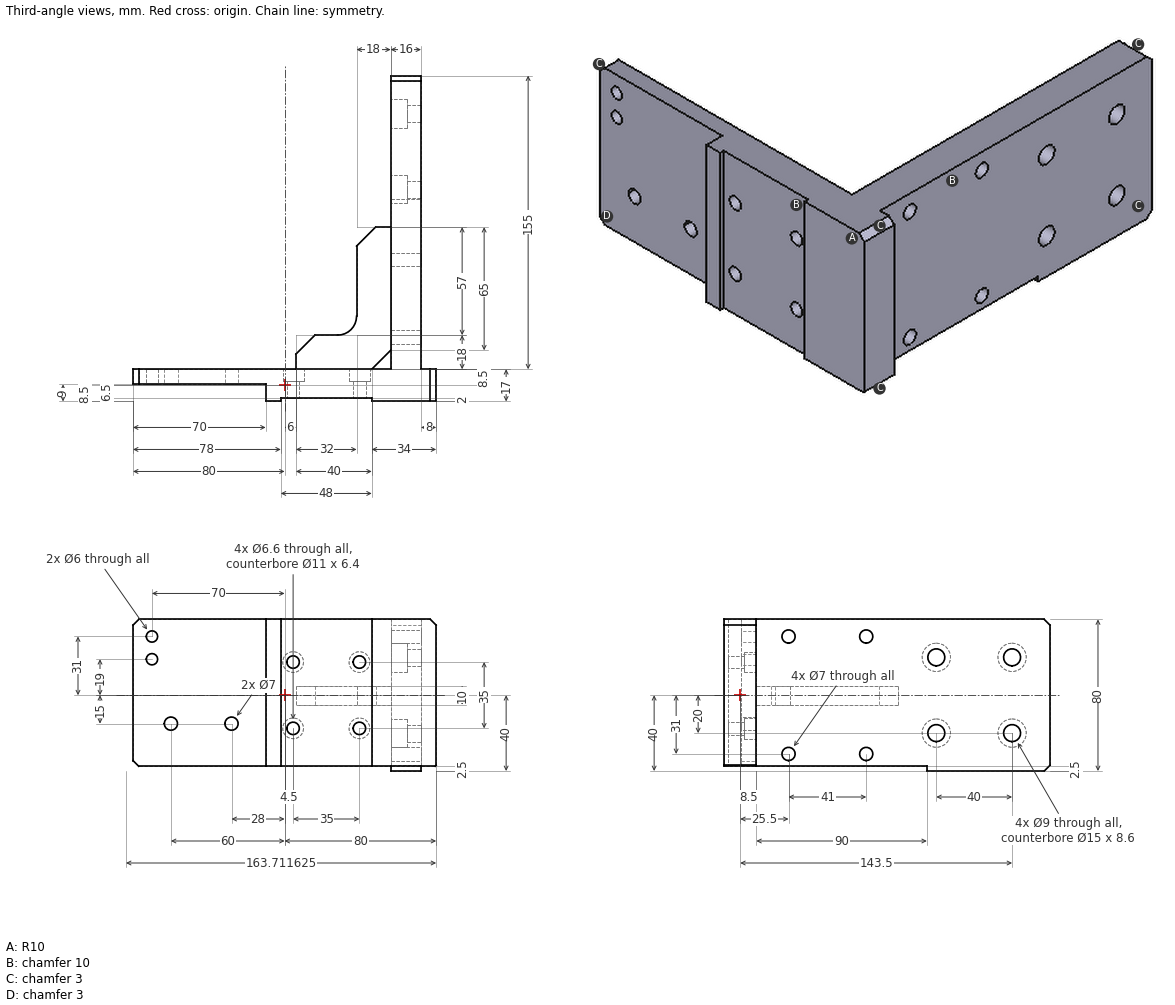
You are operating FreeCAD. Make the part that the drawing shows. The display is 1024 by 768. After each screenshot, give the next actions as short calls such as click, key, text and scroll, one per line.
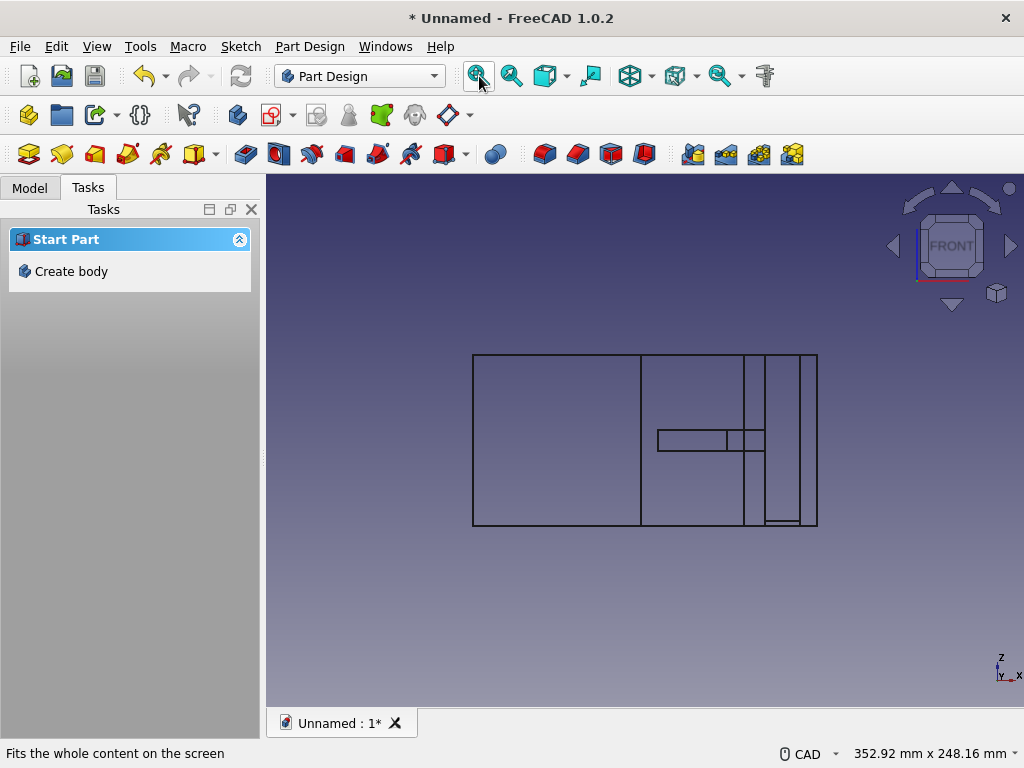
click(727, 440)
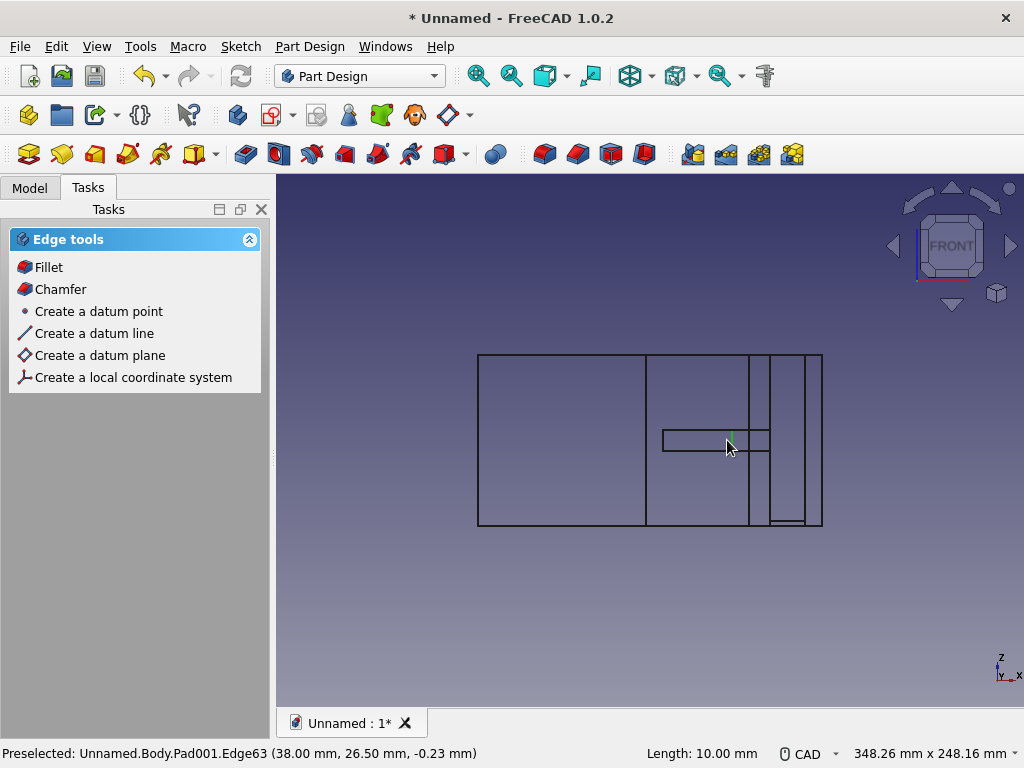
key(v)
key(1)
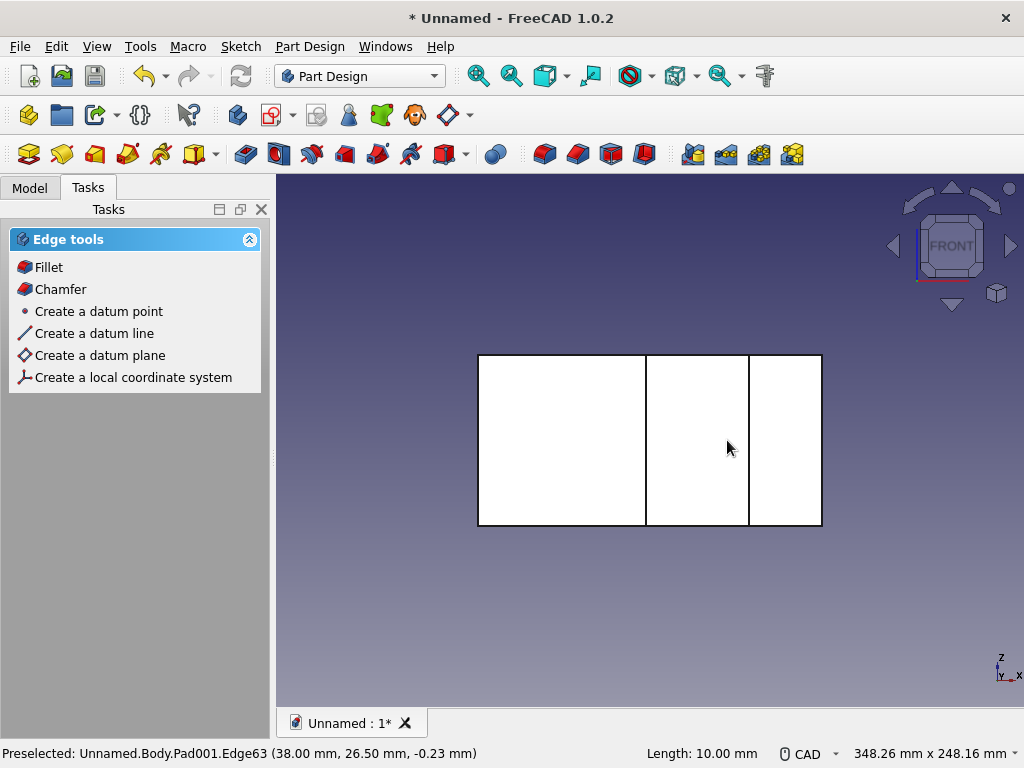
click(545, 154)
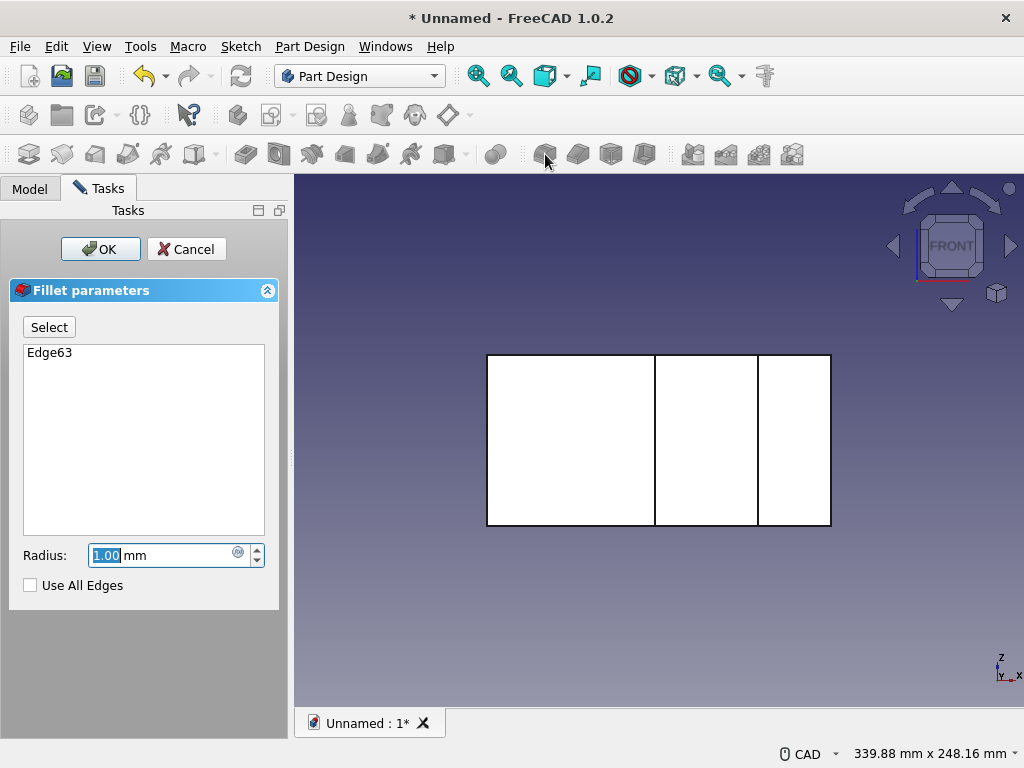
text(10)
key(Tab)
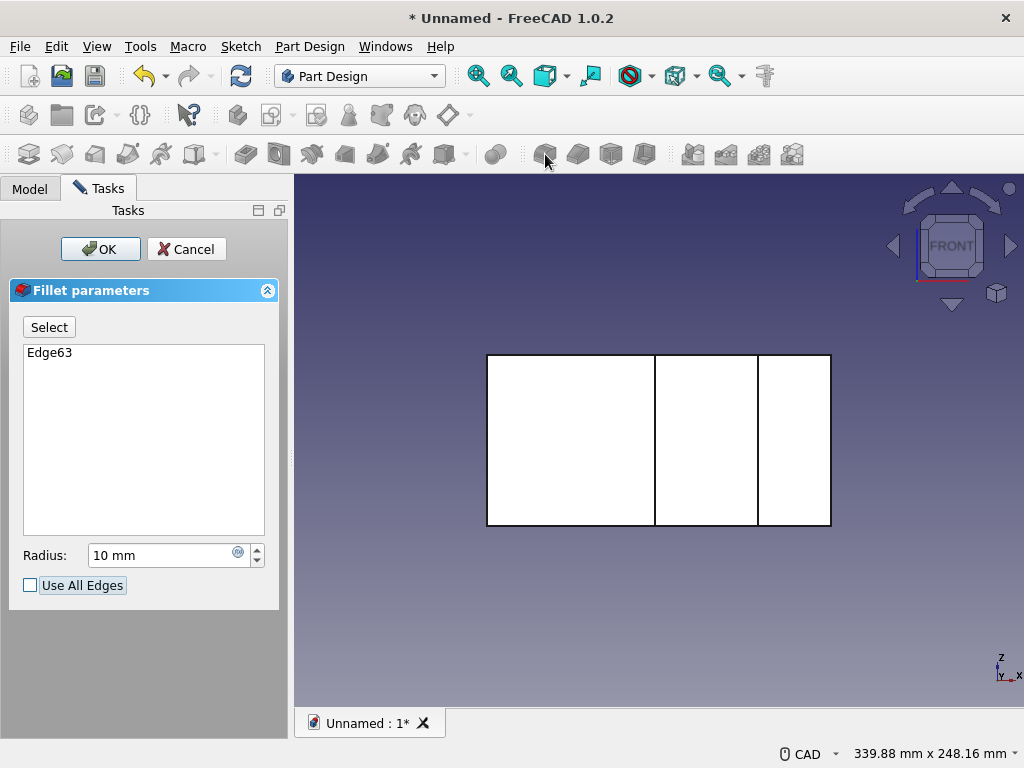
click(101, 249)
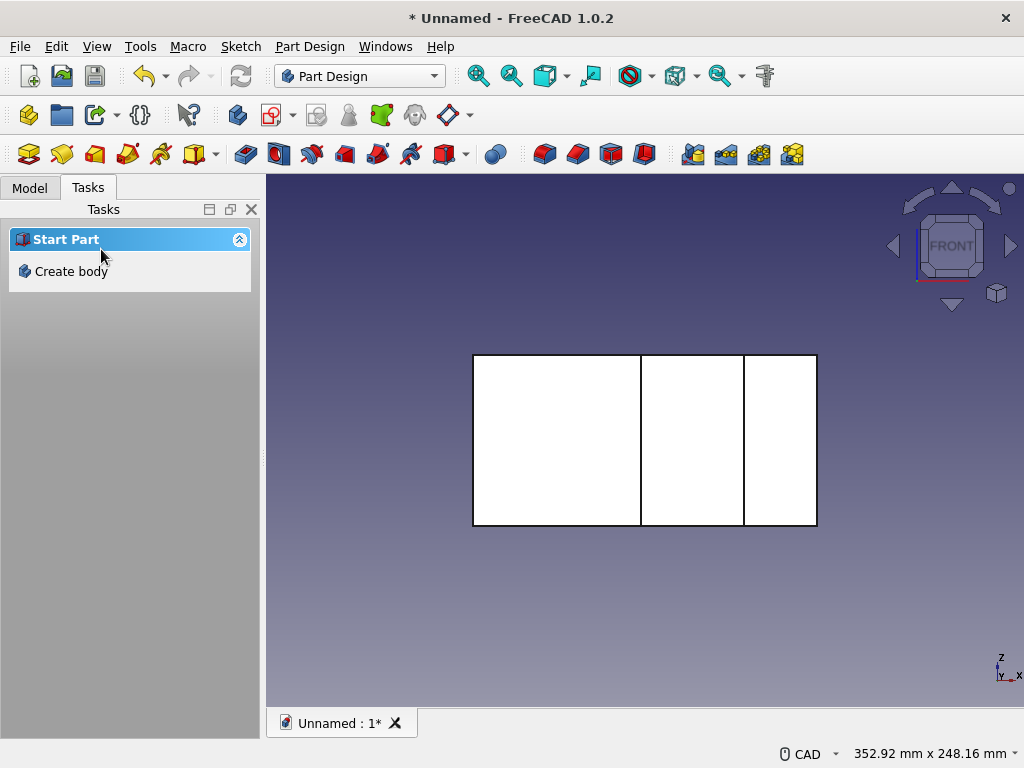
scroll(658, 440, up, 4)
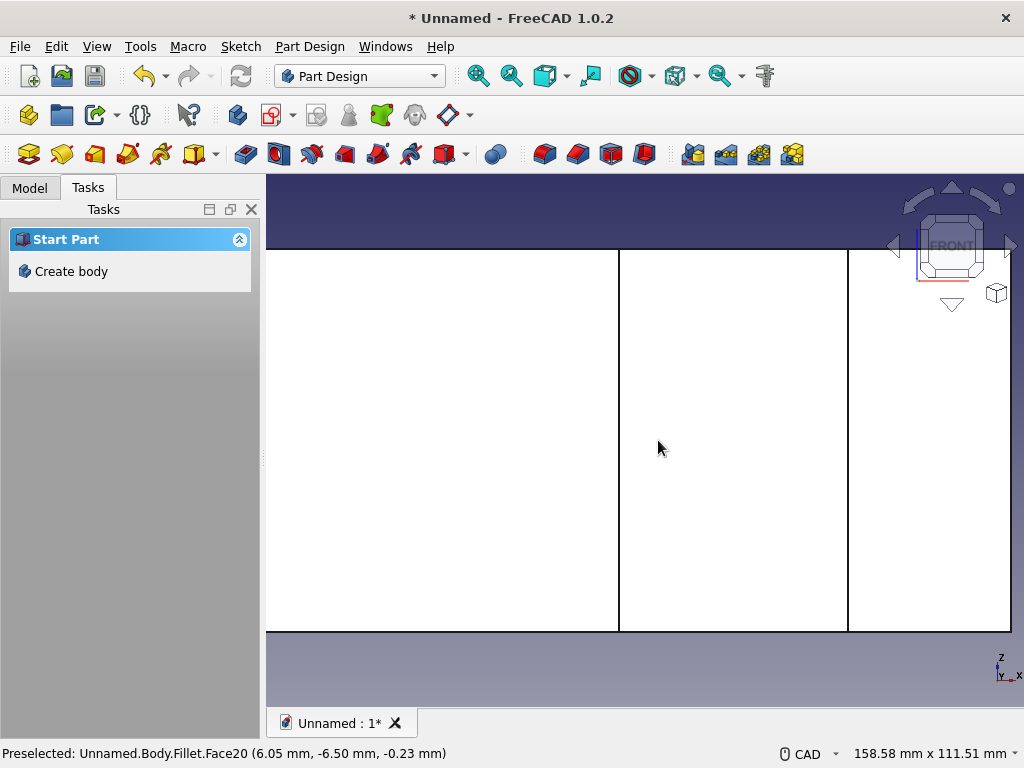
click(479, 76)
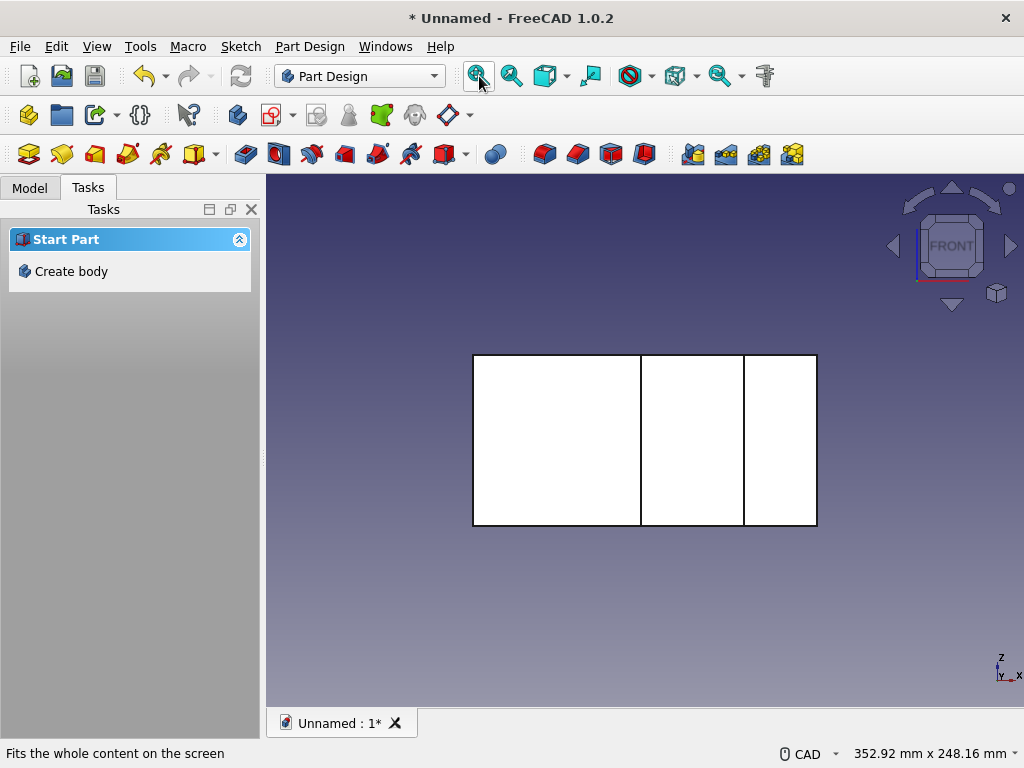
key(0)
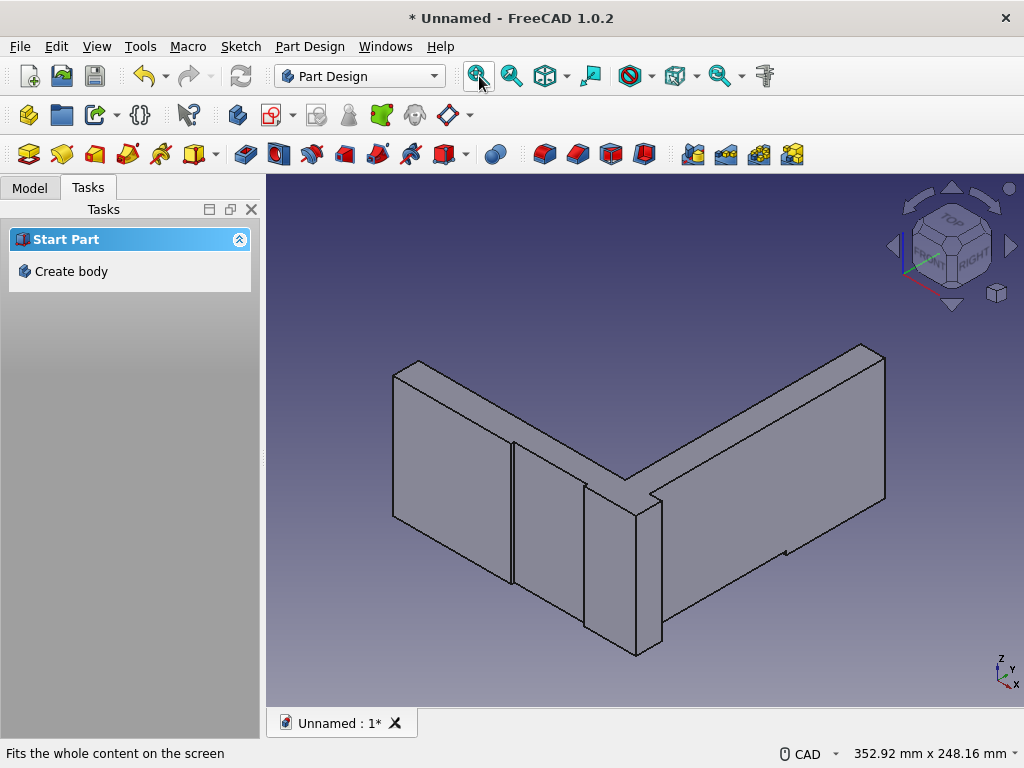
scroll(577, 489, up, 4)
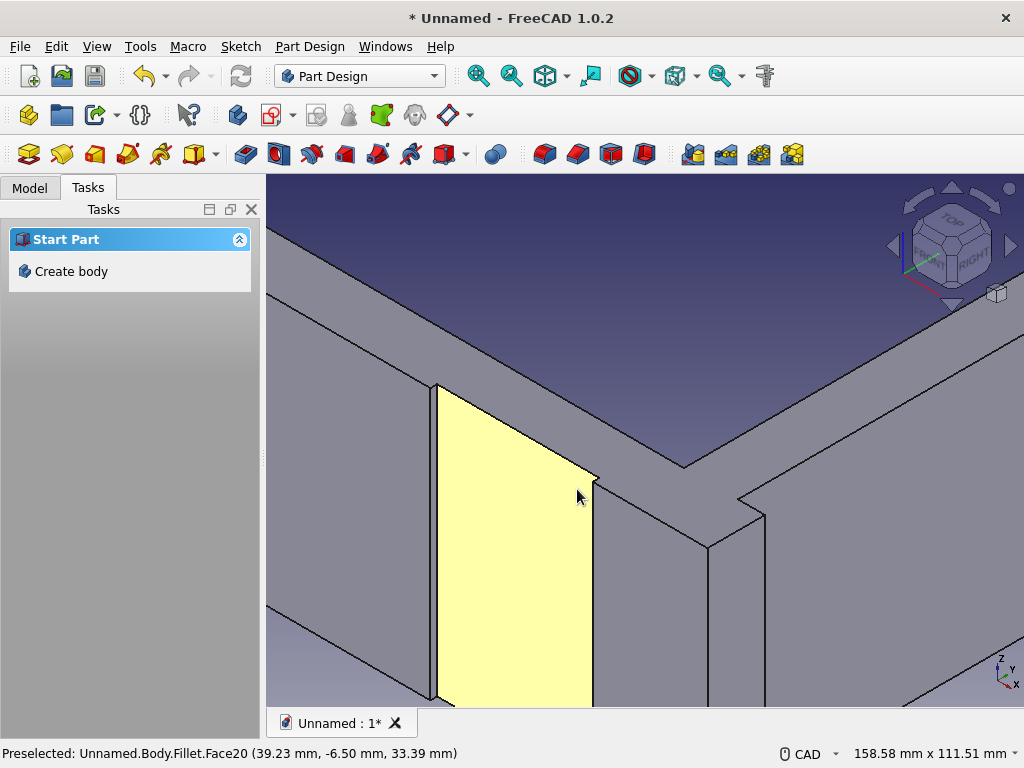
click(479, 76)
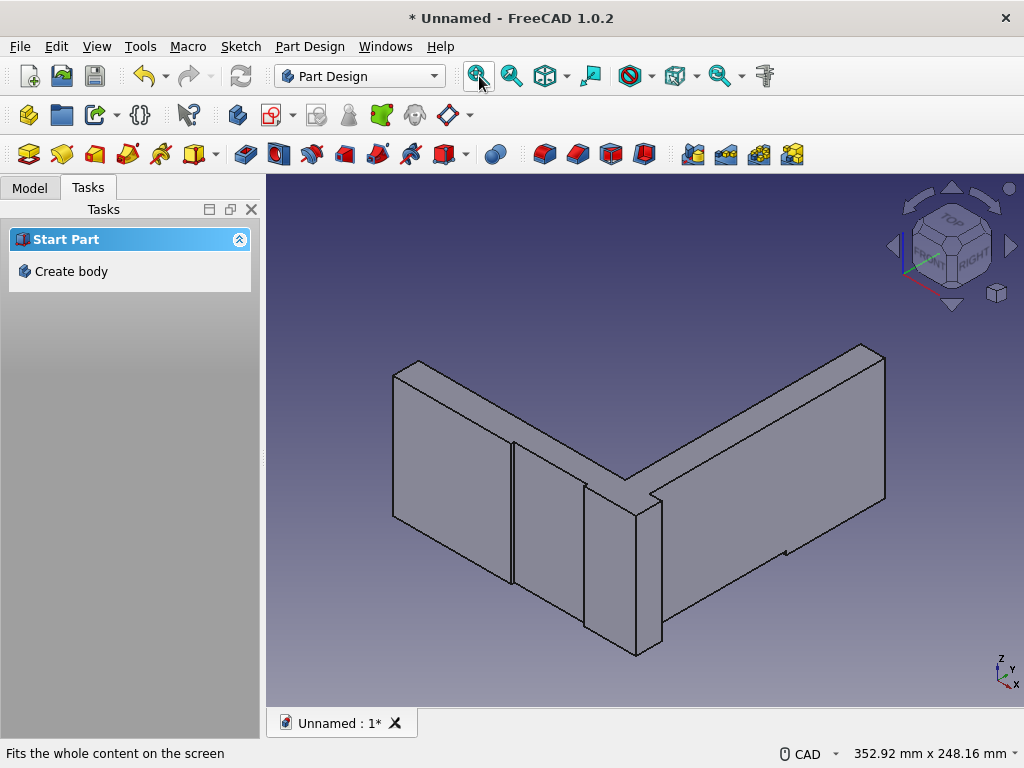
key(2)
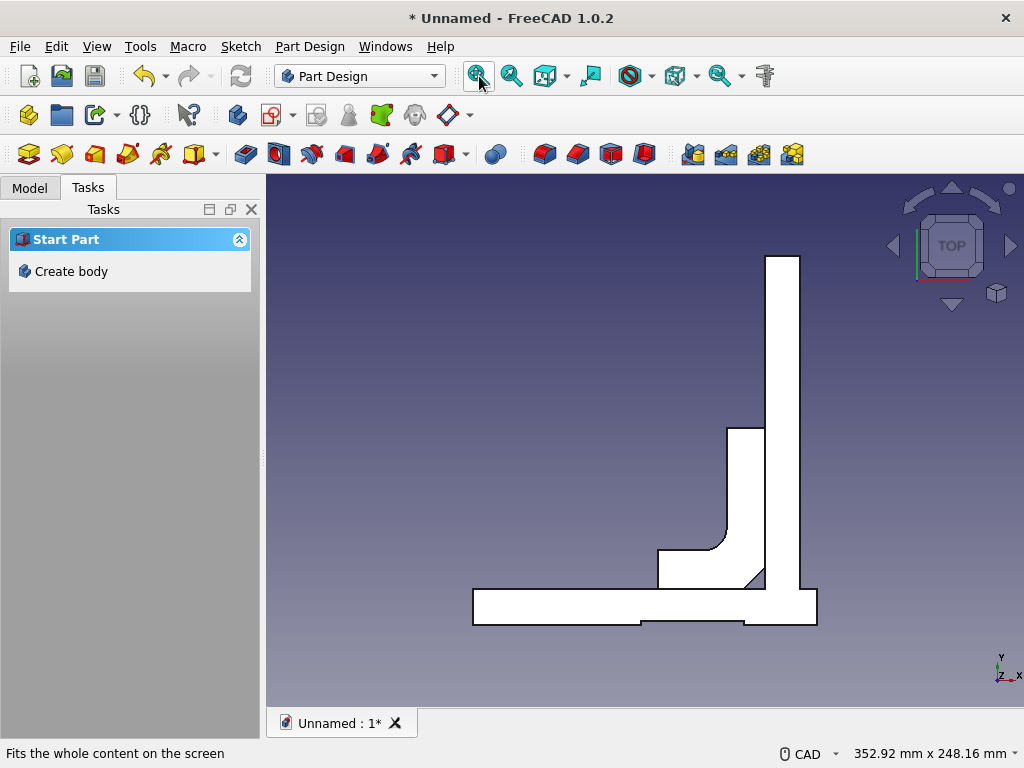
scroll(658, 549, up, 4)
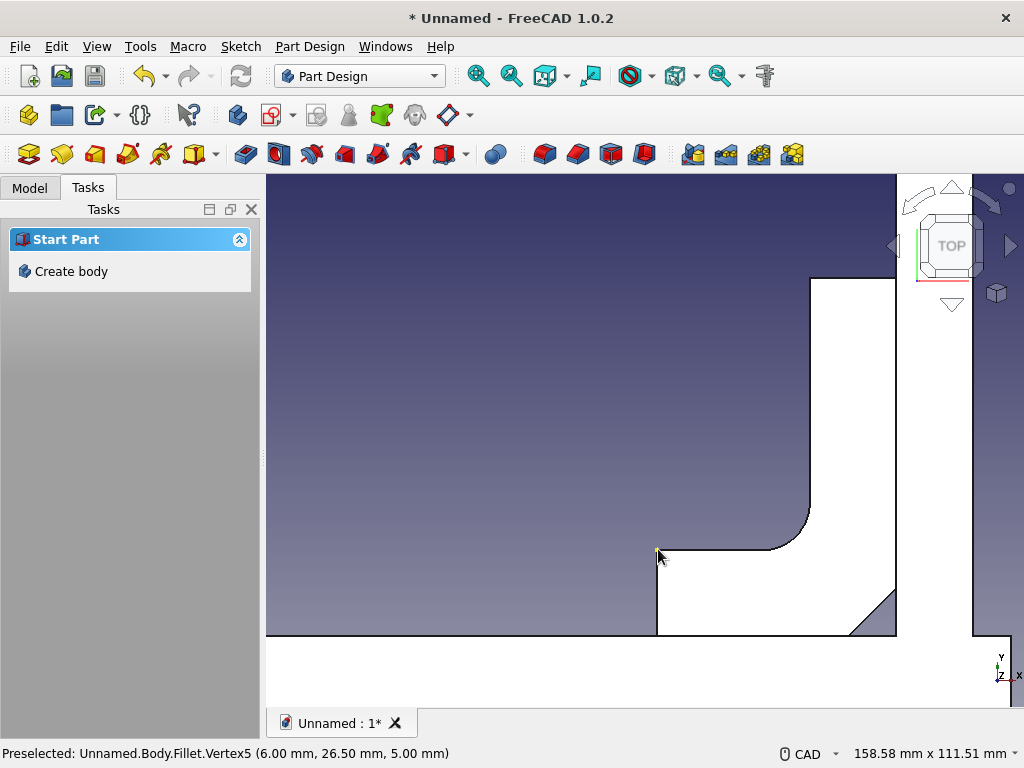
click(479, 76)